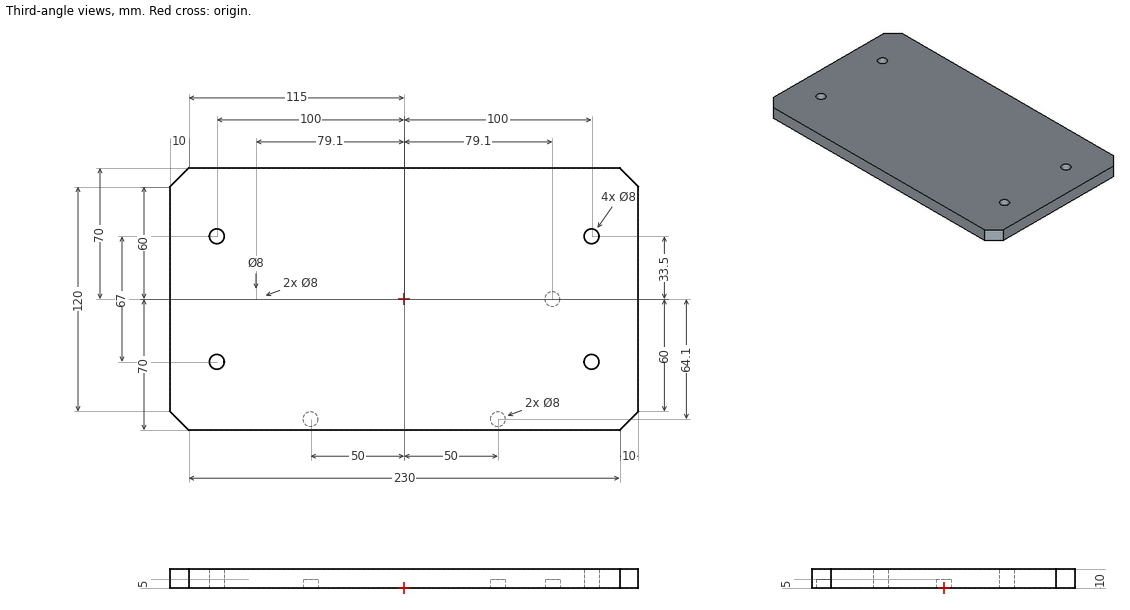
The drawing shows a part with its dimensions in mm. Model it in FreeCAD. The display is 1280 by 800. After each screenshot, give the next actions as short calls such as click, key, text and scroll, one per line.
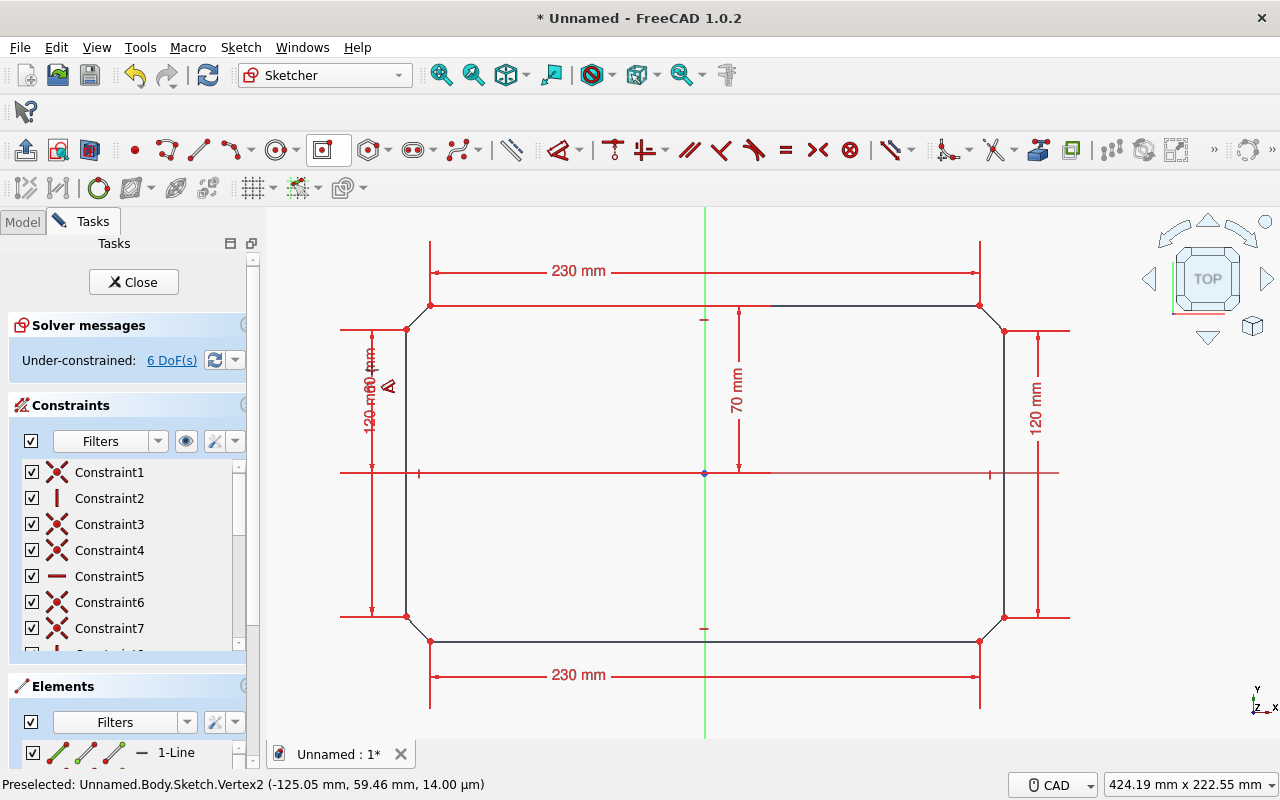
click(430, 642)
click(739, 558)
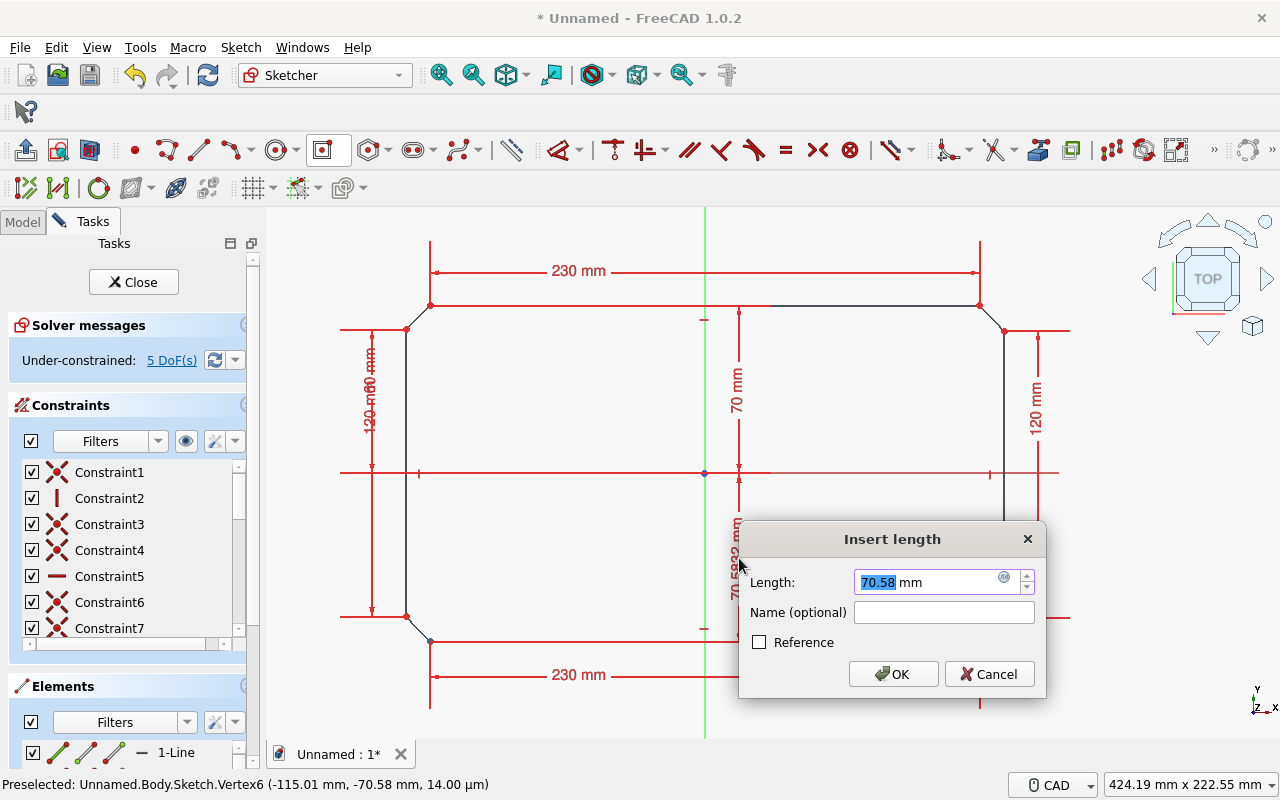
text(70)
key(Return)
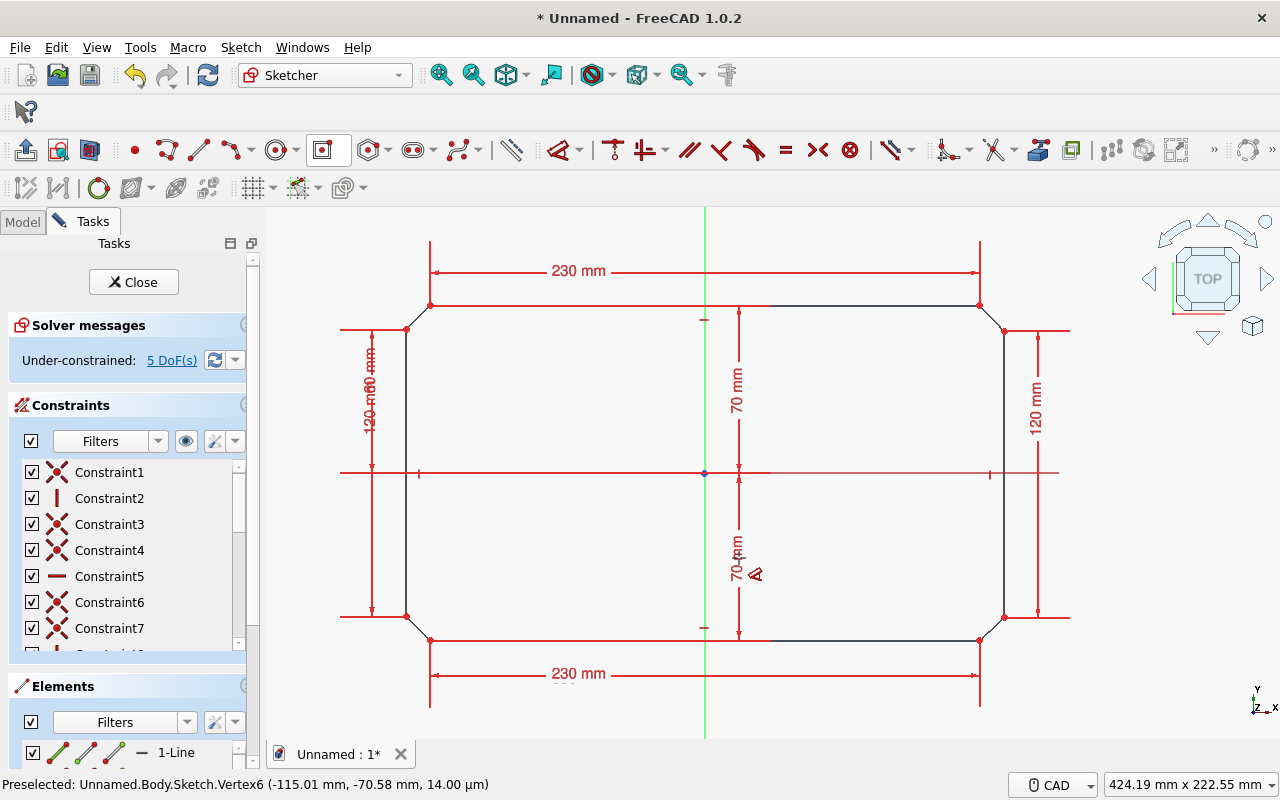
click(1004, 618)
click(1038, 546)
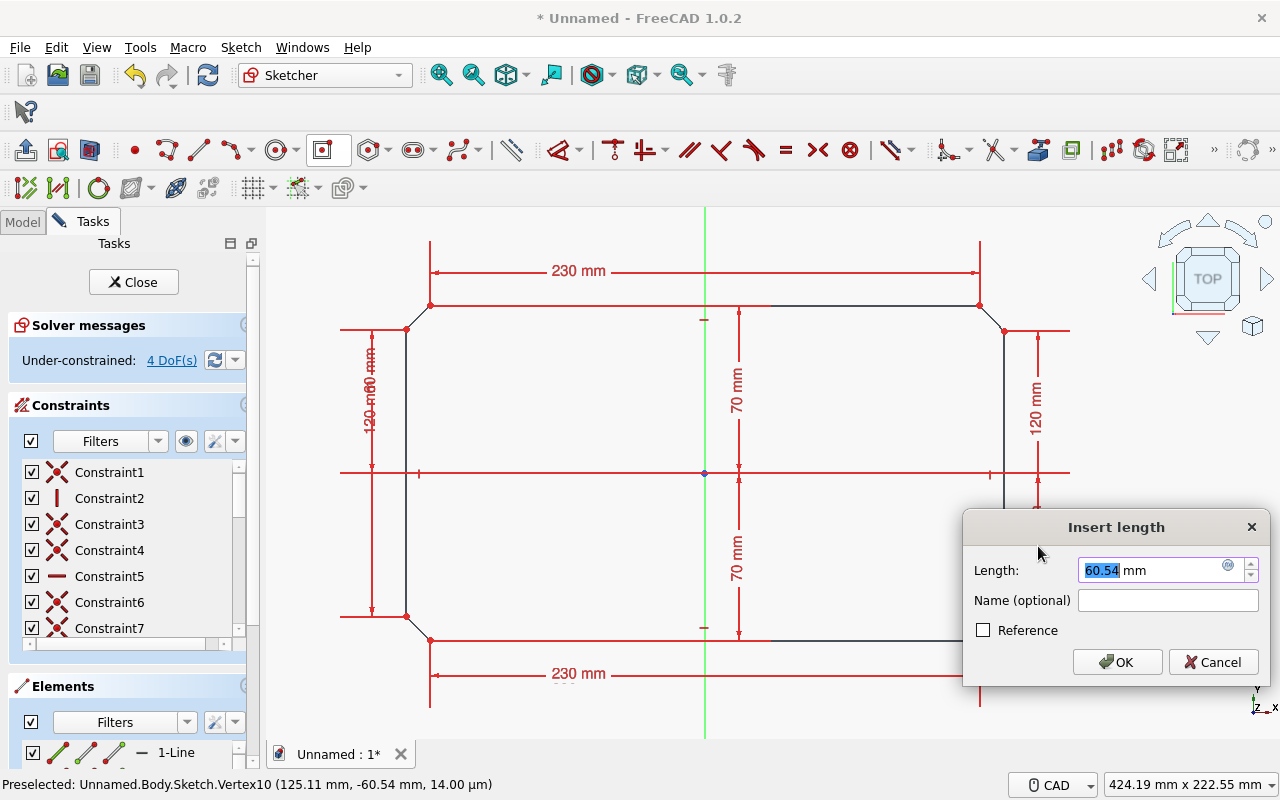
text(60)
key(Return)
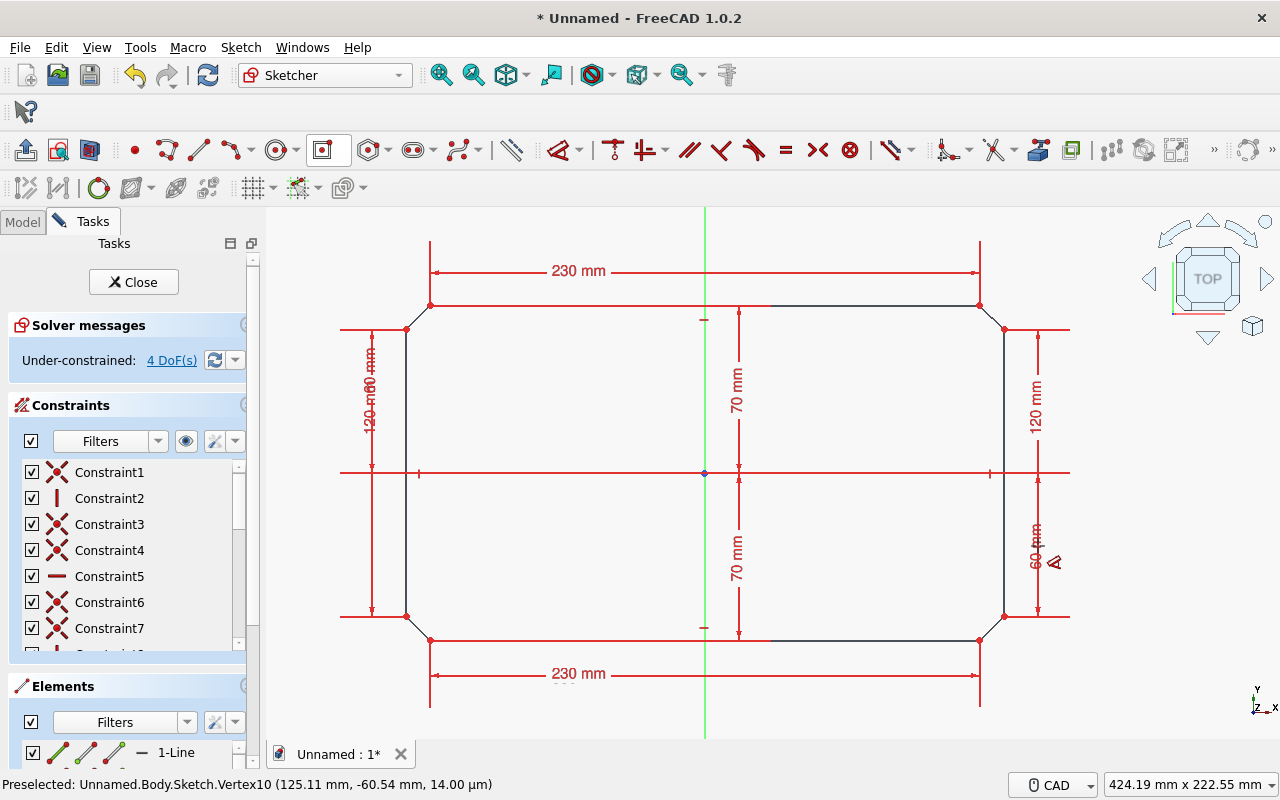
scroll(423, 313, up, 3)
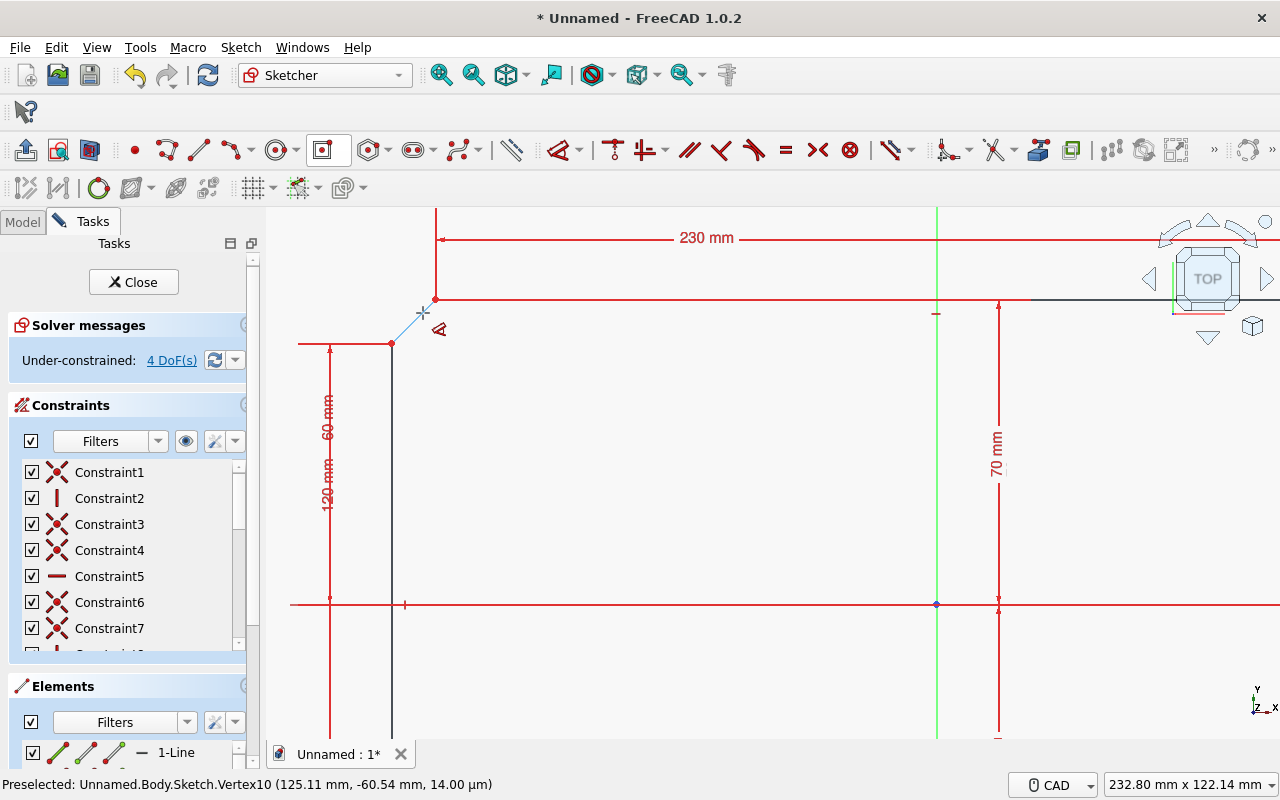
click(423, 313)
click(414, 266)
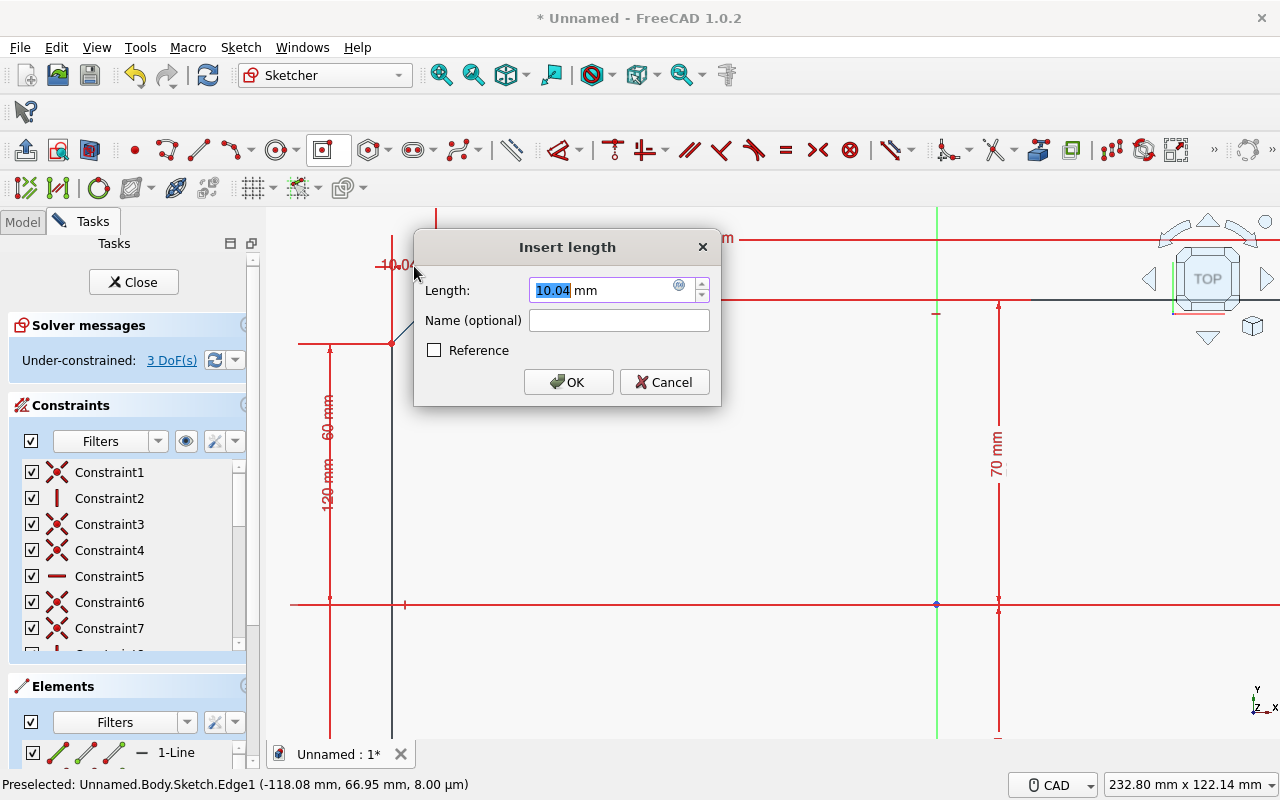
text(10)
key(Return)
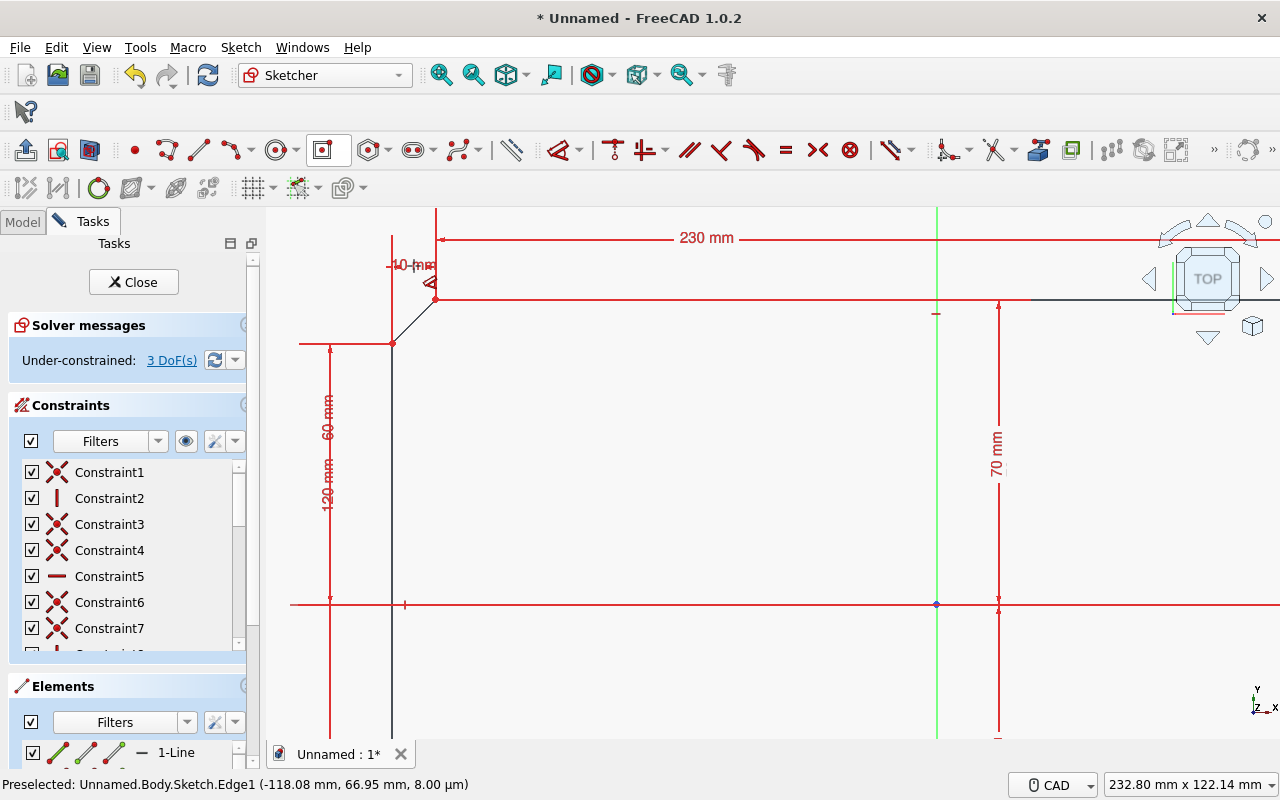
scroll(422, 313, down, 3)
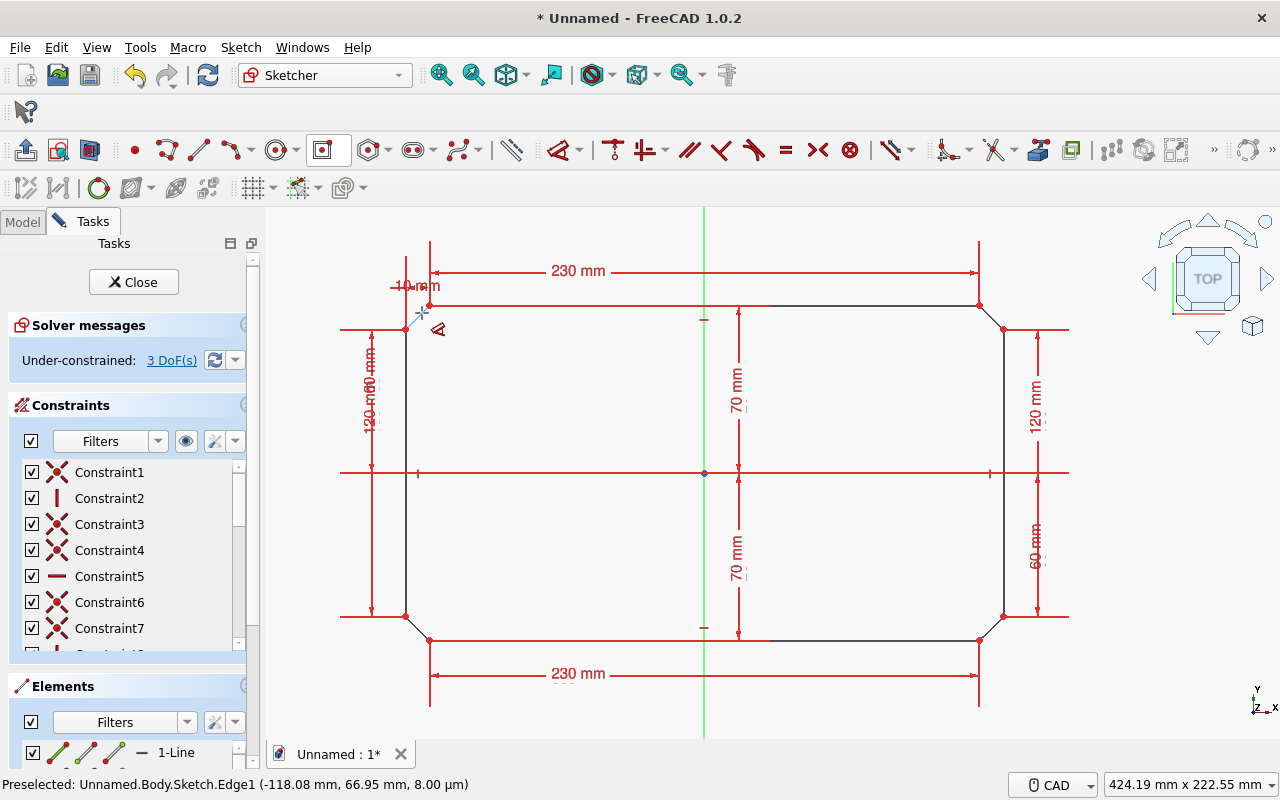
scroll(413, 624, up, 3)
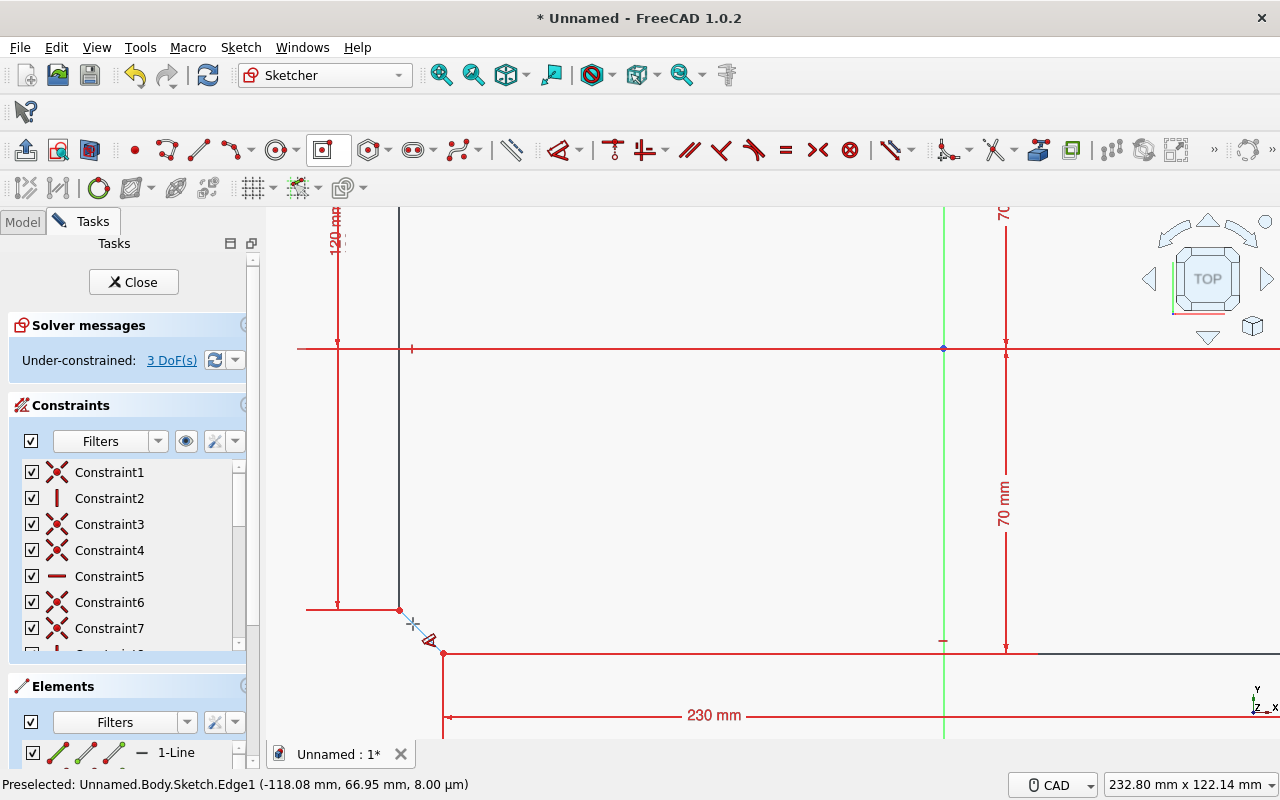
click(413, 623)
click(421, 688)